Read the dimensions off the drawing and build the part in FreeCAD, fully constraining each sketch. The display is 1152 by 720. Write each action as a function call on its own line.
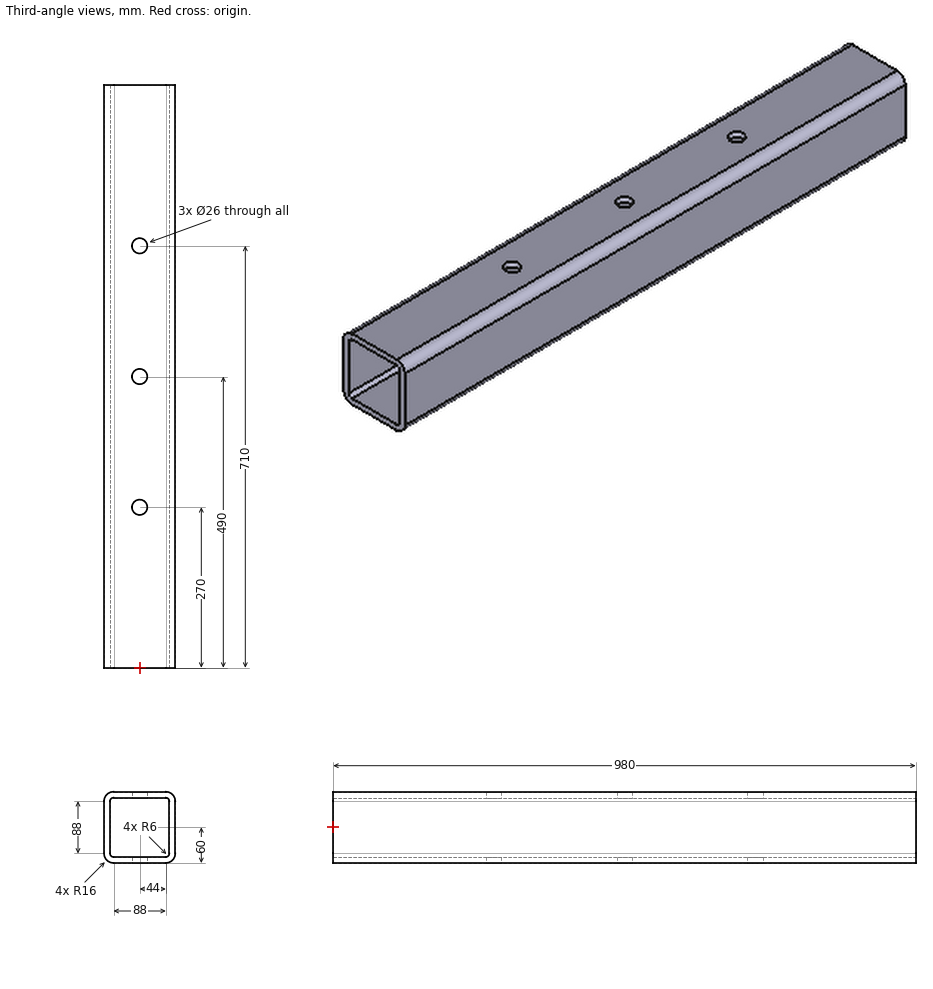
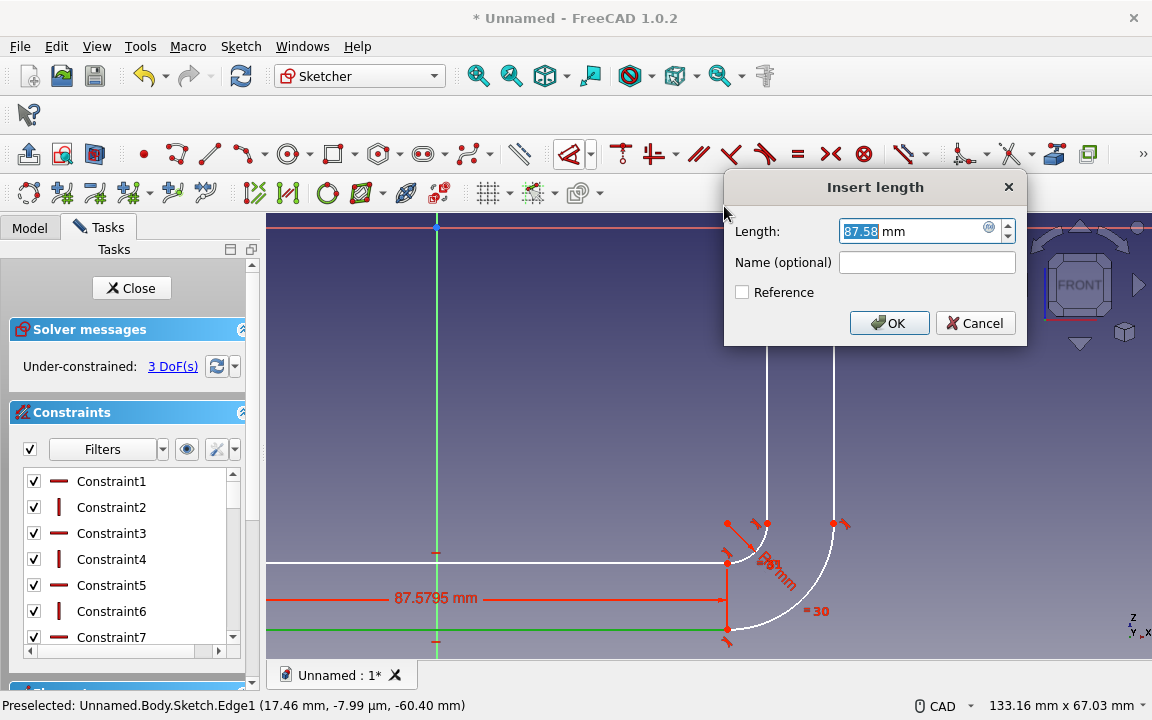
text(88)
key(Return)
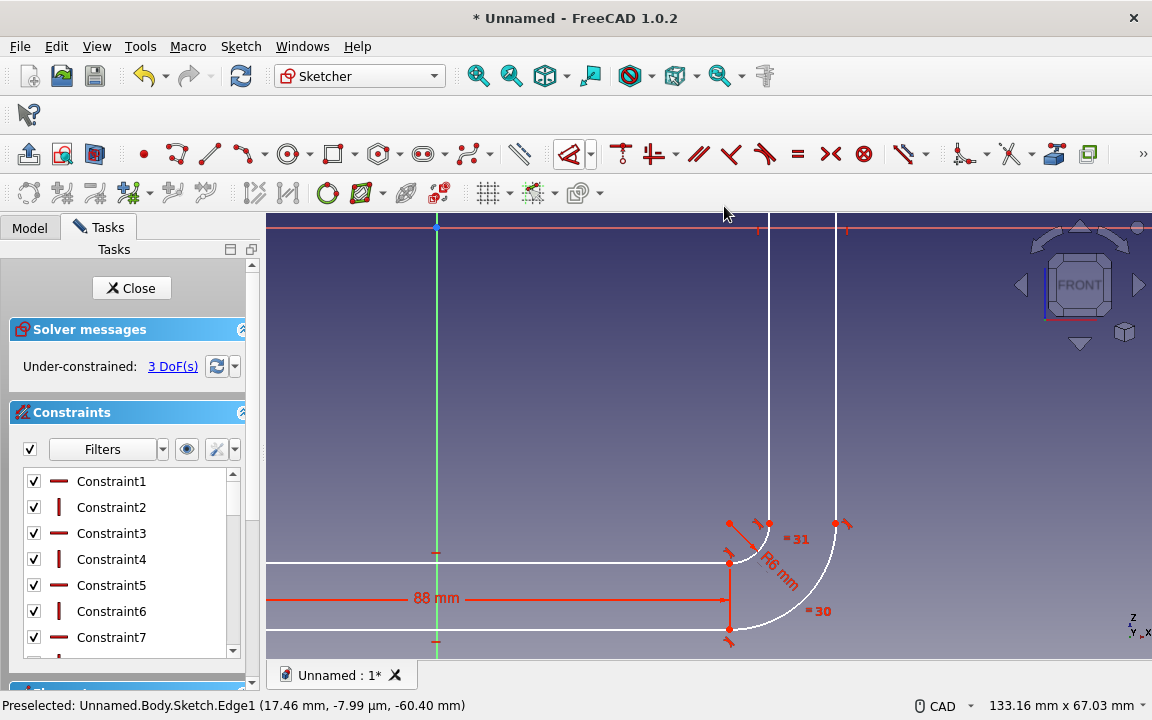
scroll(759, 557, down, 5)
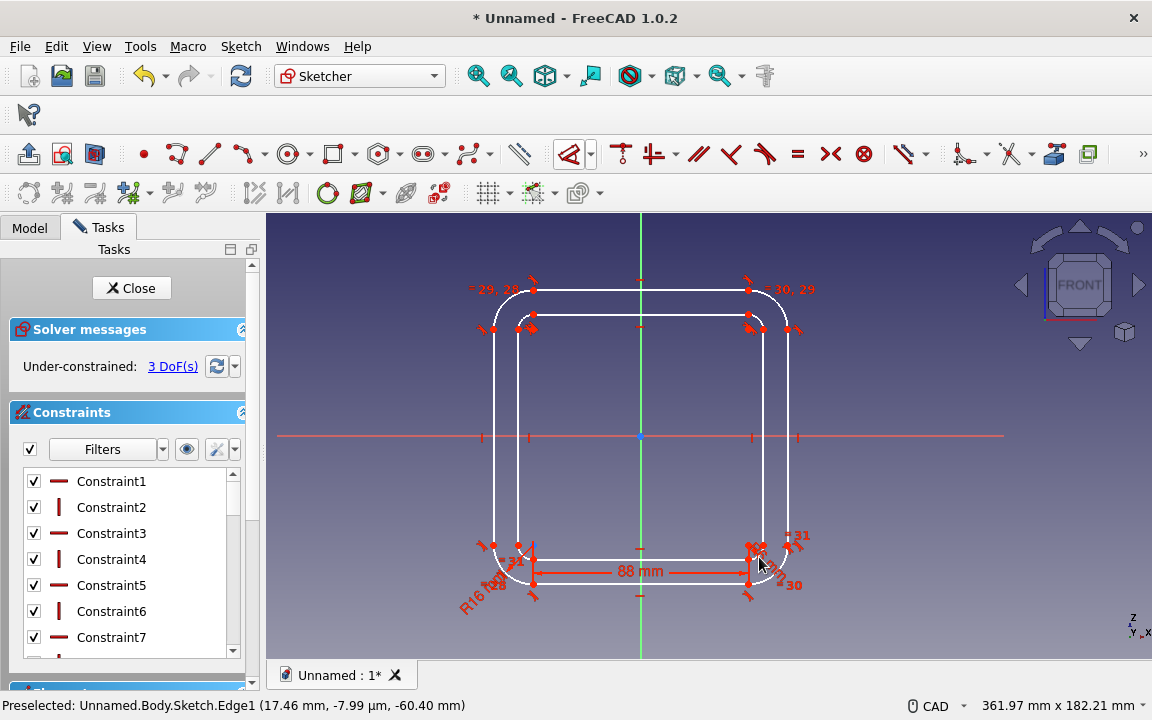
click(494, 480)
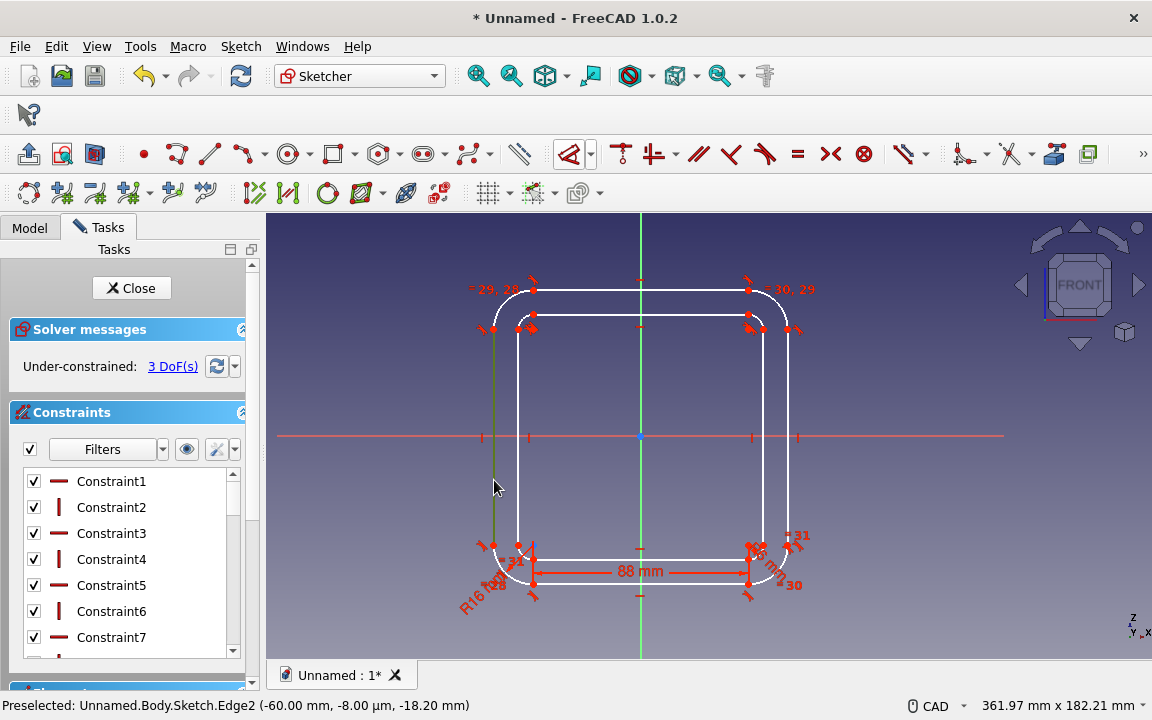
key(i)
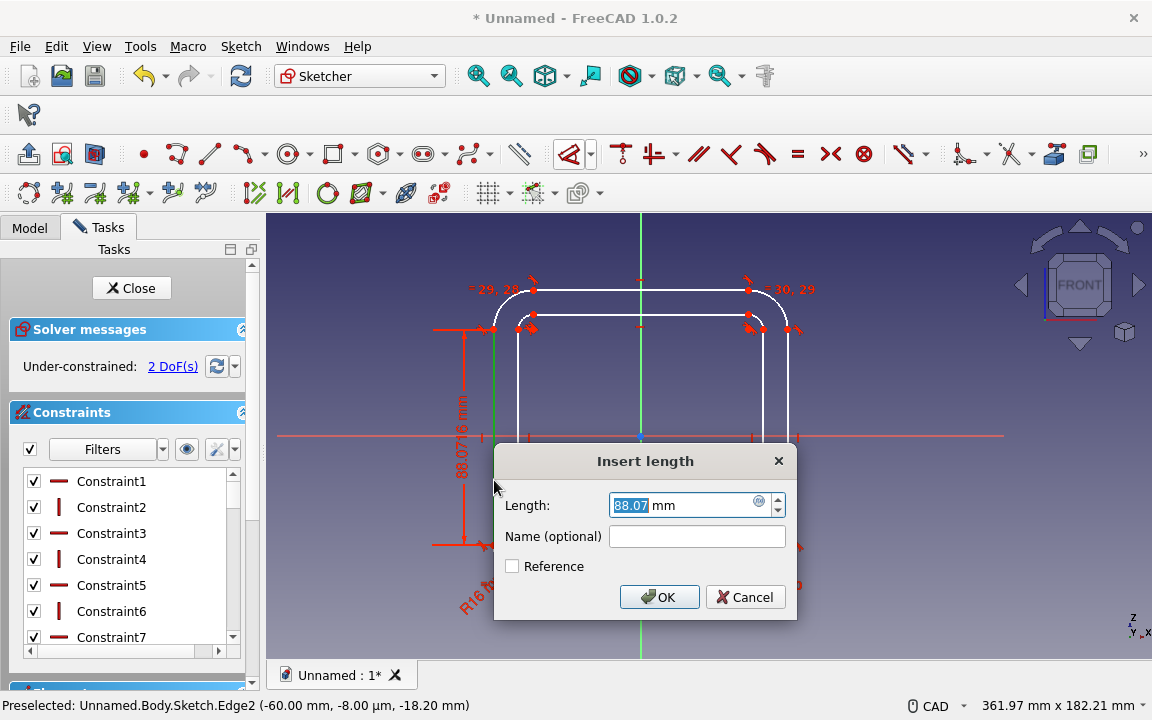
text(88)
key(Return)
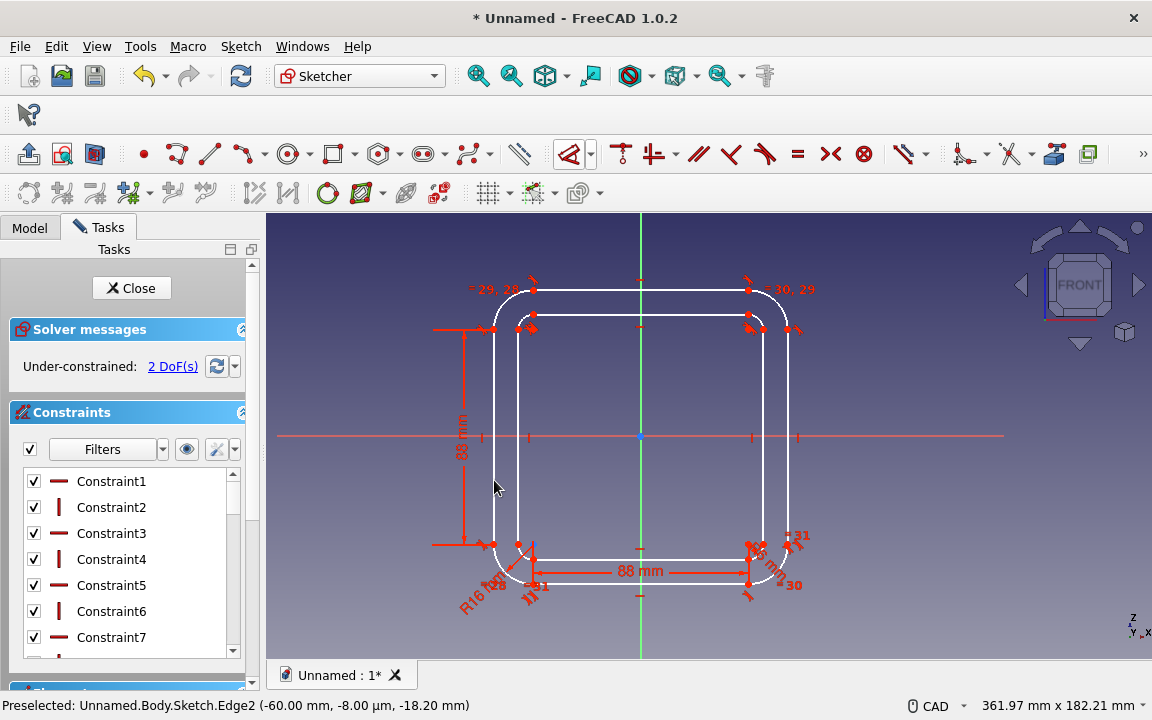
click(749, 584)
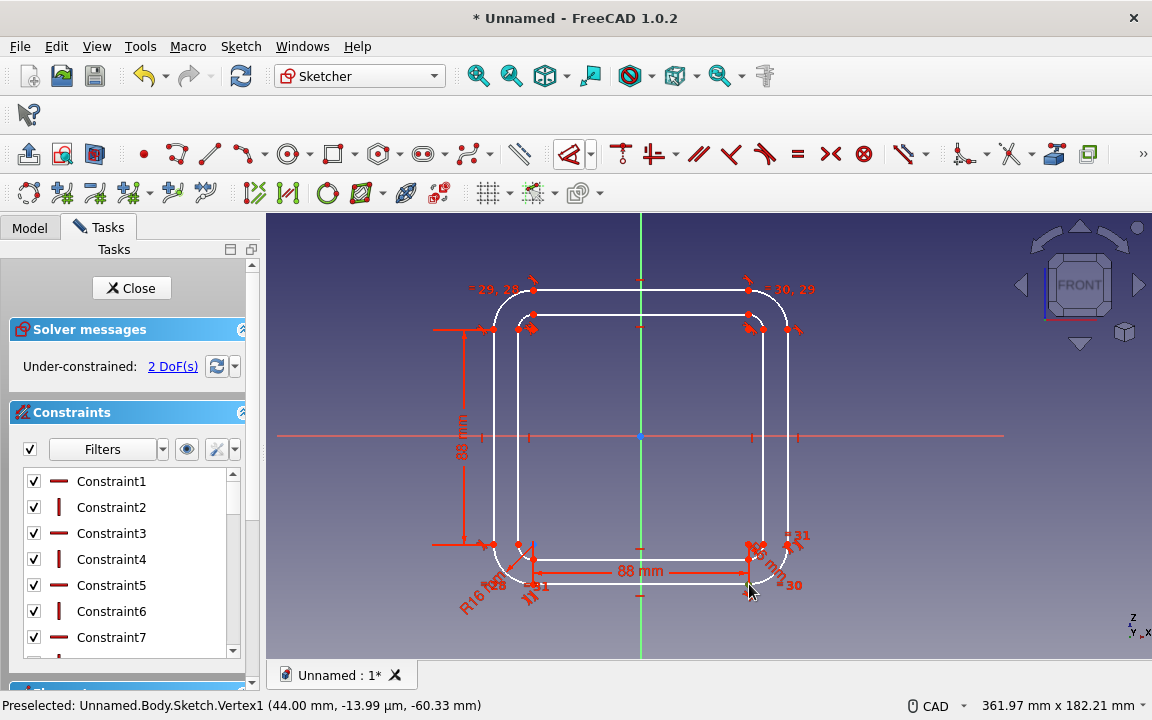
key(l)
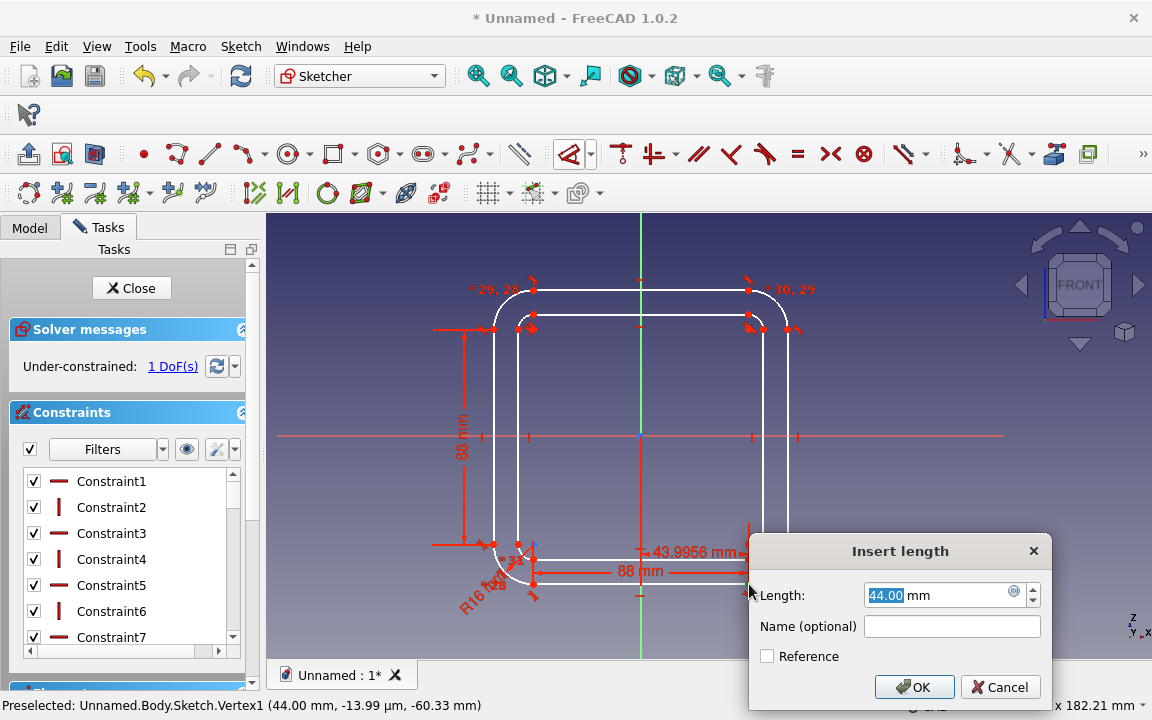
text(44)
key(Return)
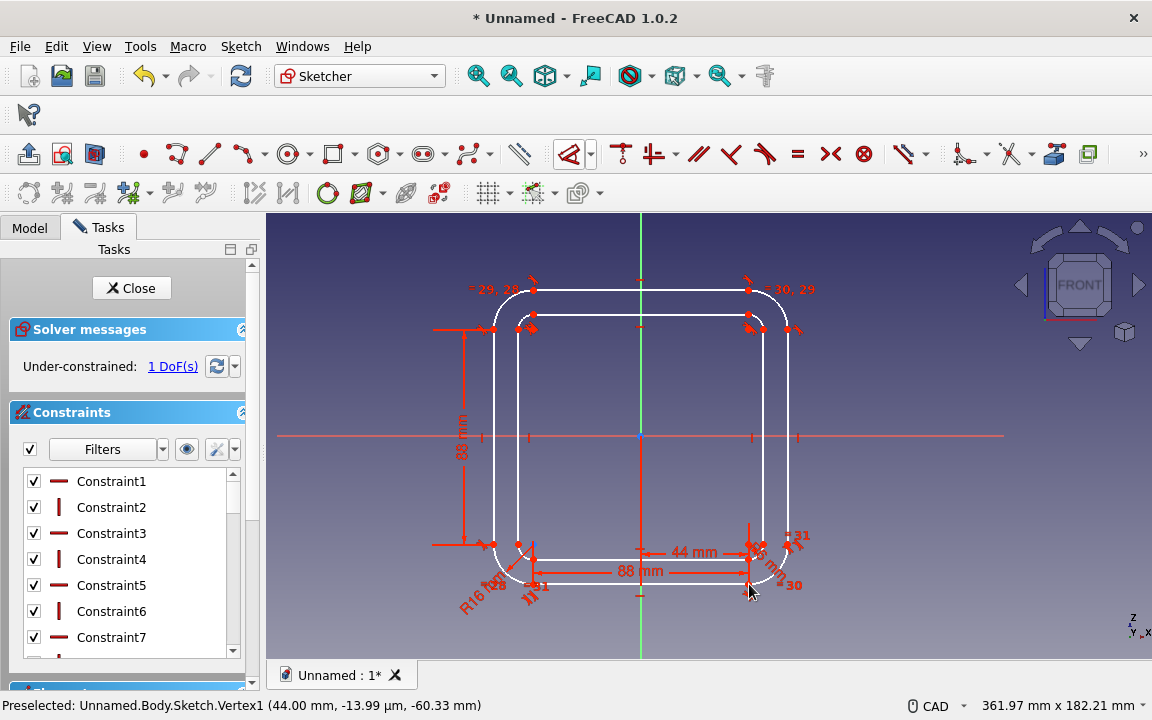
click(749, 584)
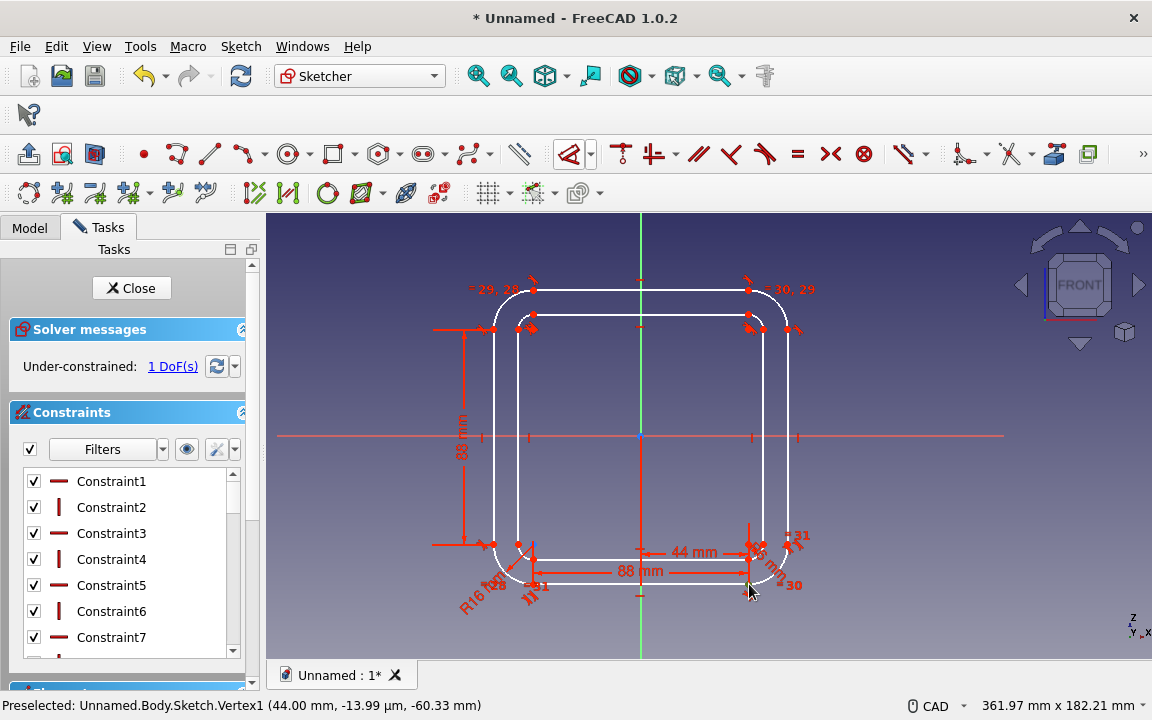
key(i)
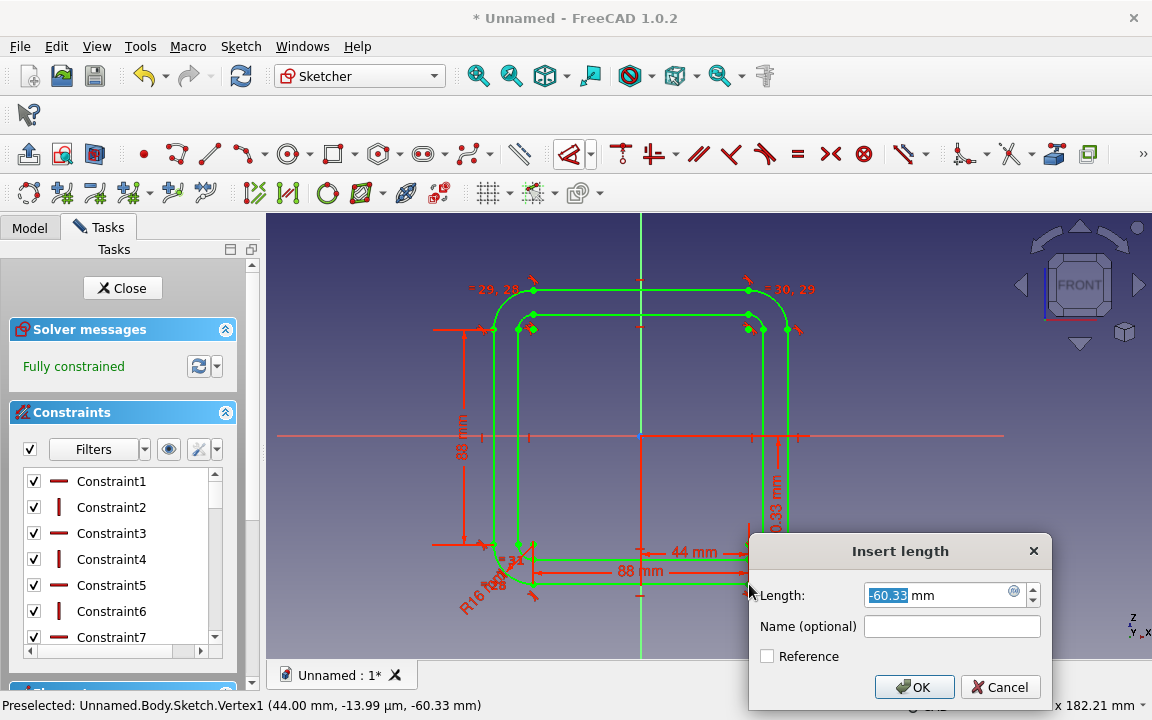
text(-60)
key(Return)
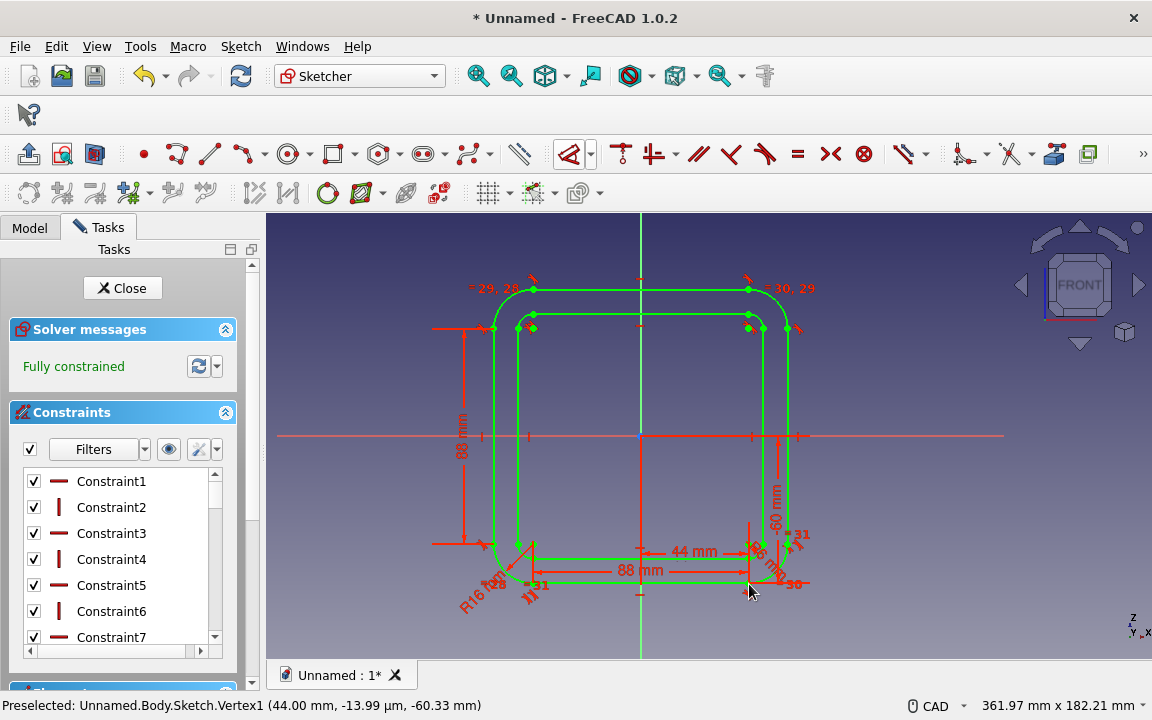
click(123, 288)